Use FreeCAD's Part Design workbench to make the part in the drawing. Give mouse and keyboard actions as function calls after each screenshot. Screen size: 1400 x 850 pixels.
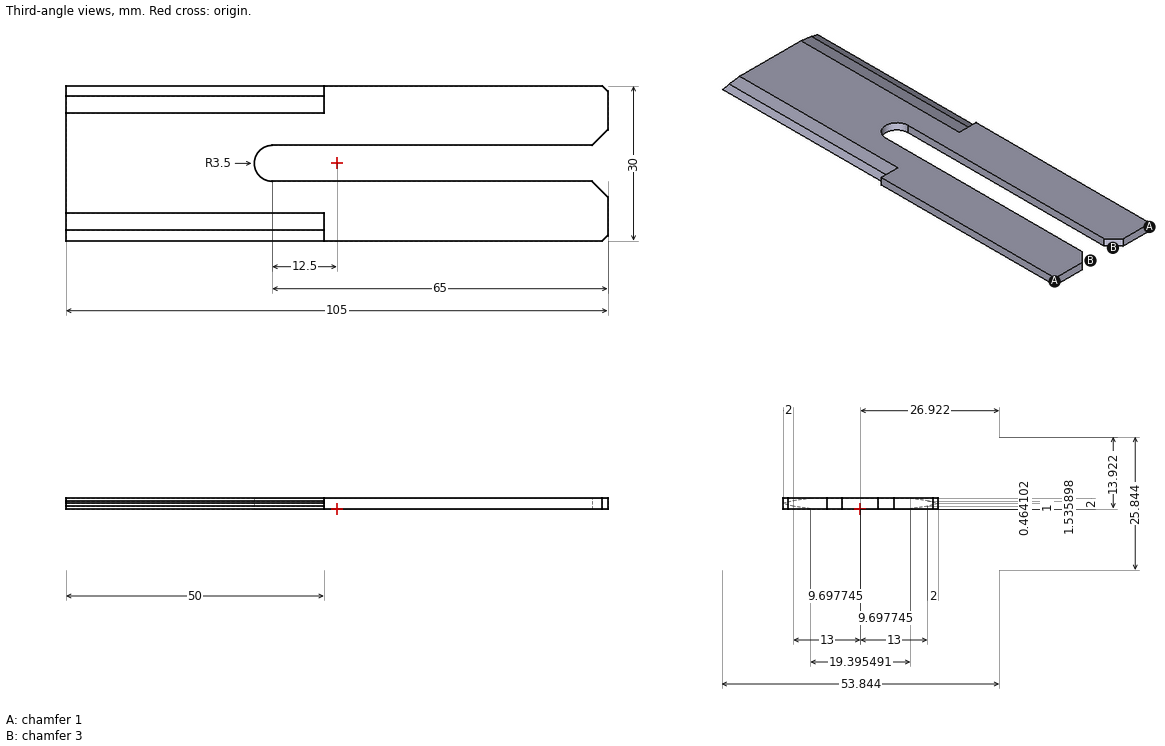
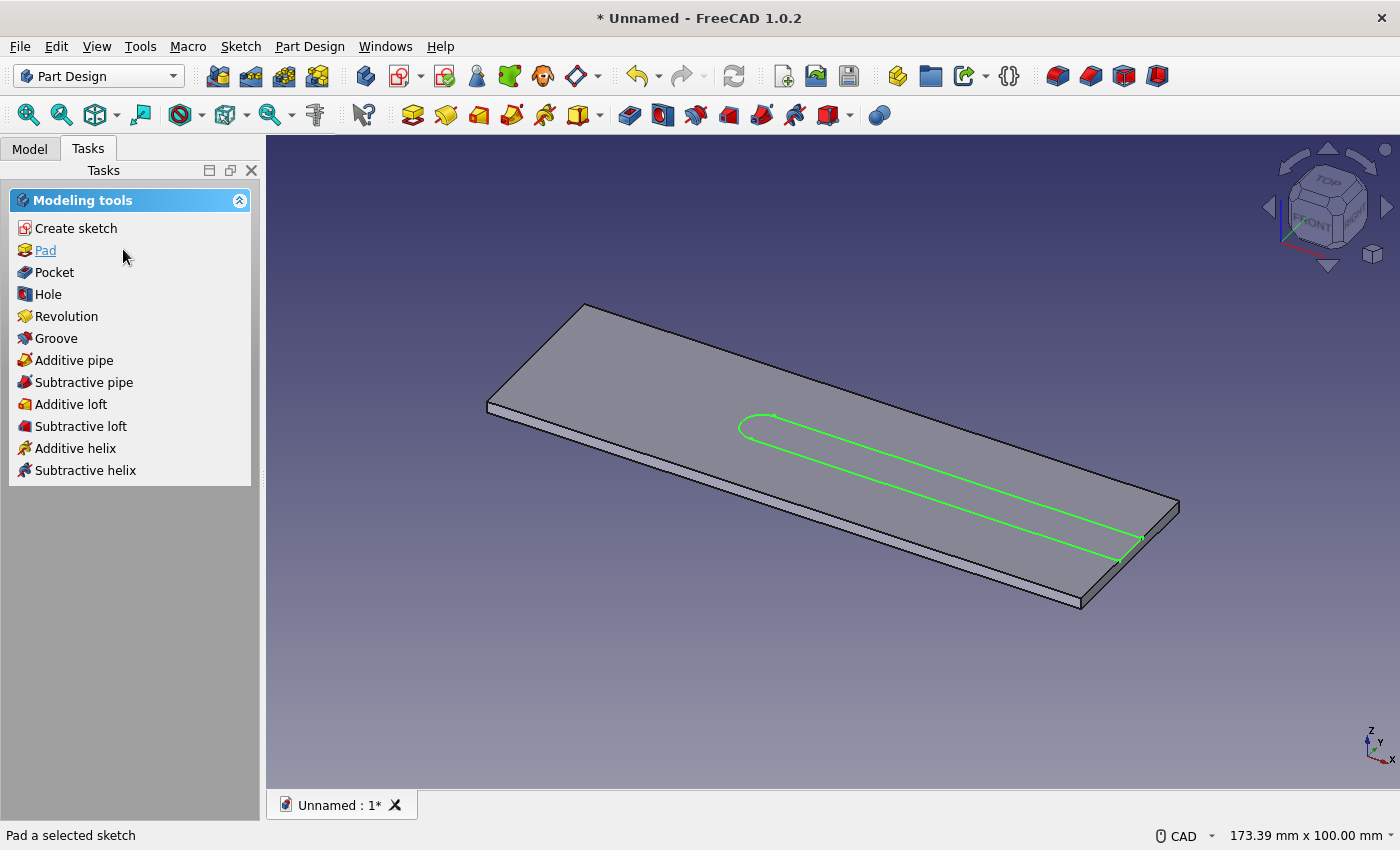
click(630, 116)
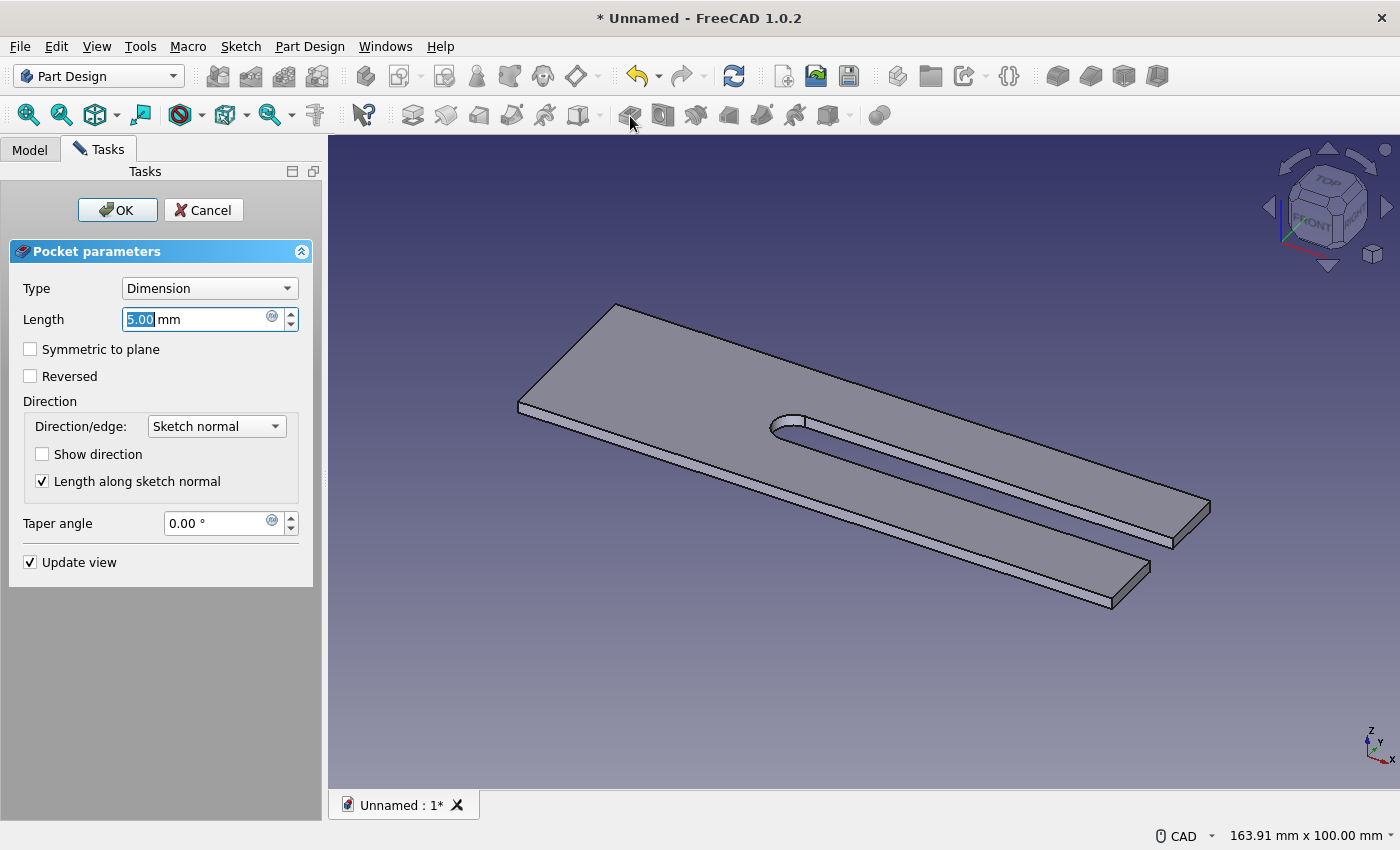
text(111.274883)
key(Tab)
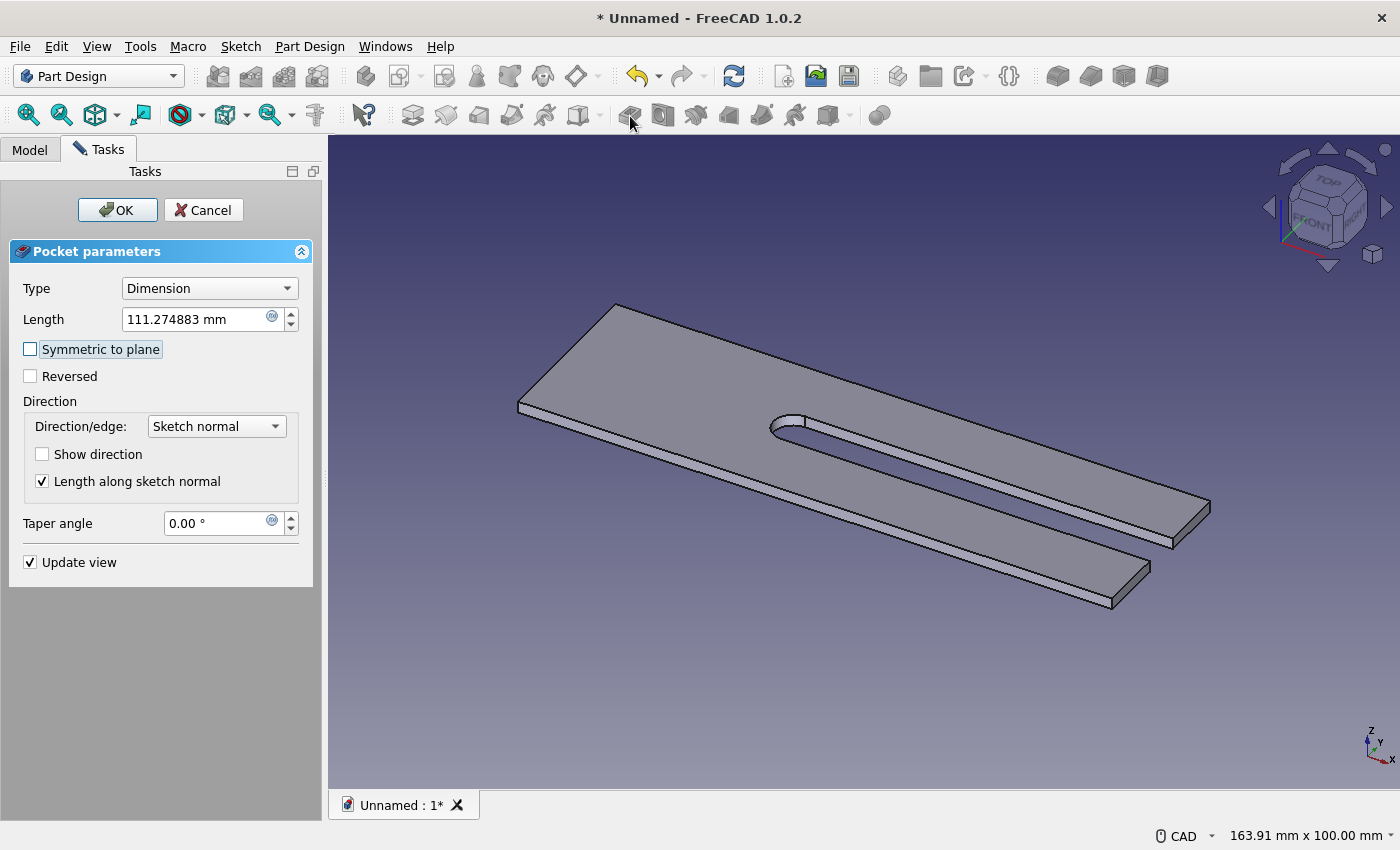
click(31, 349)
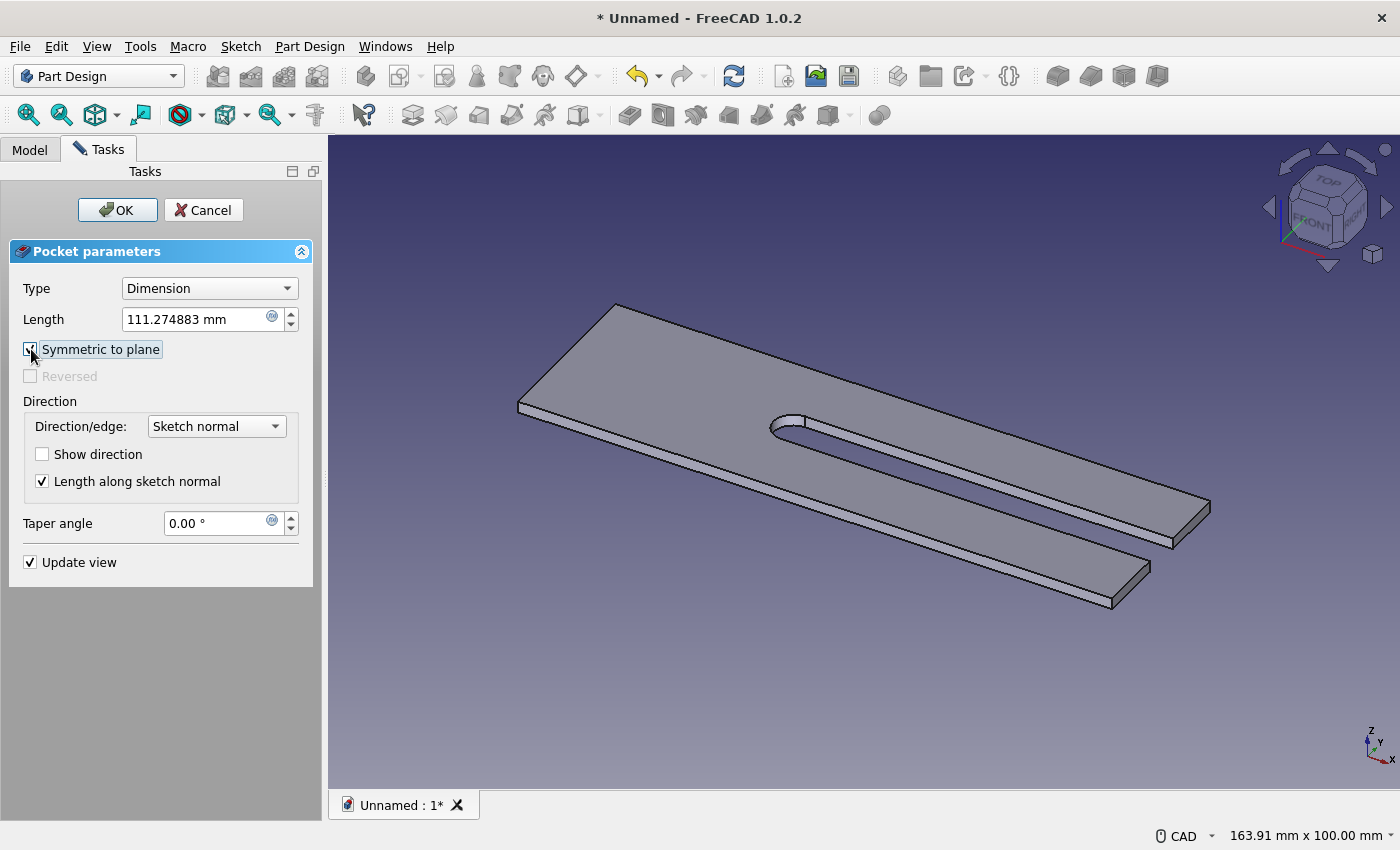
click(118, 210)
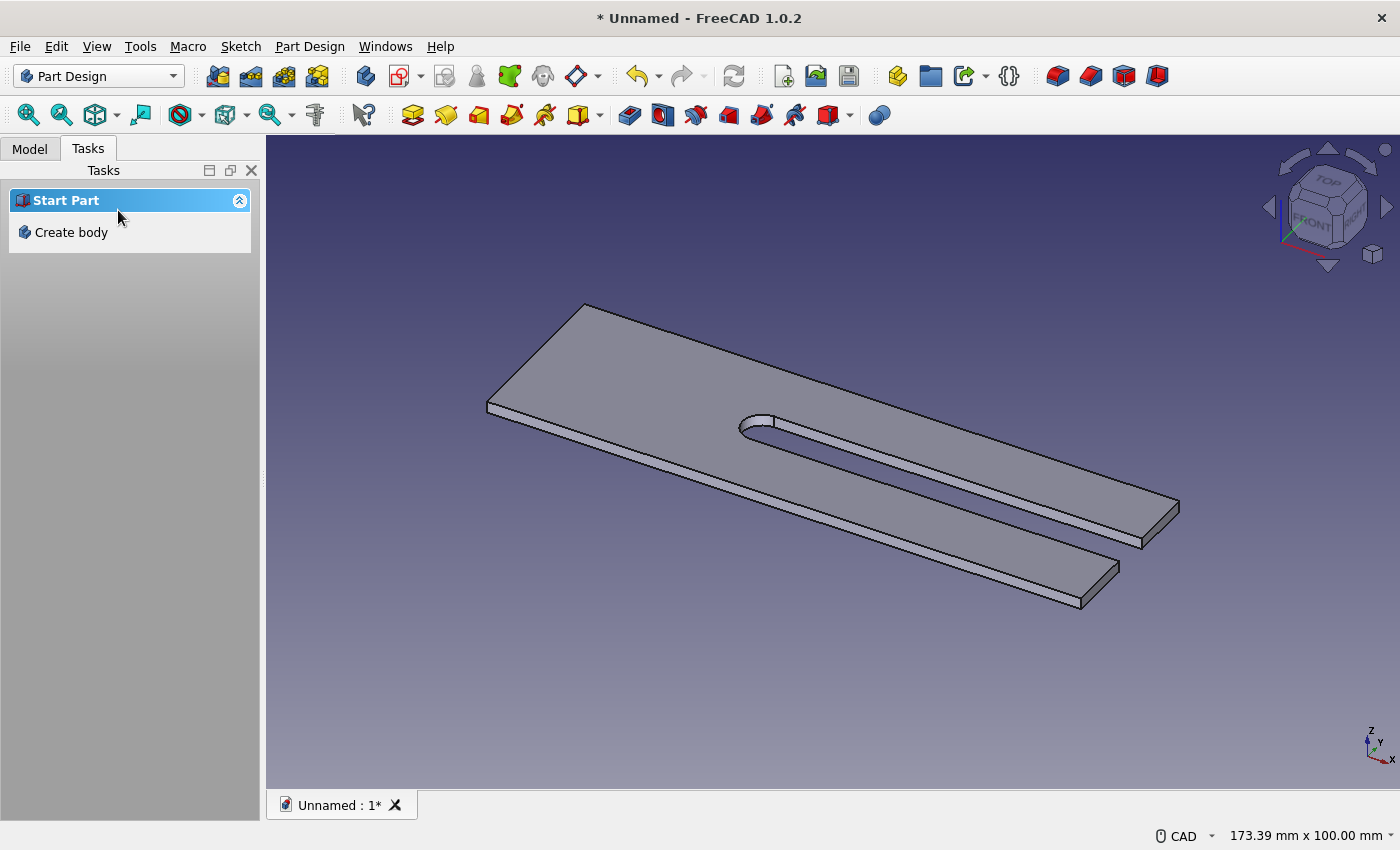
key(6)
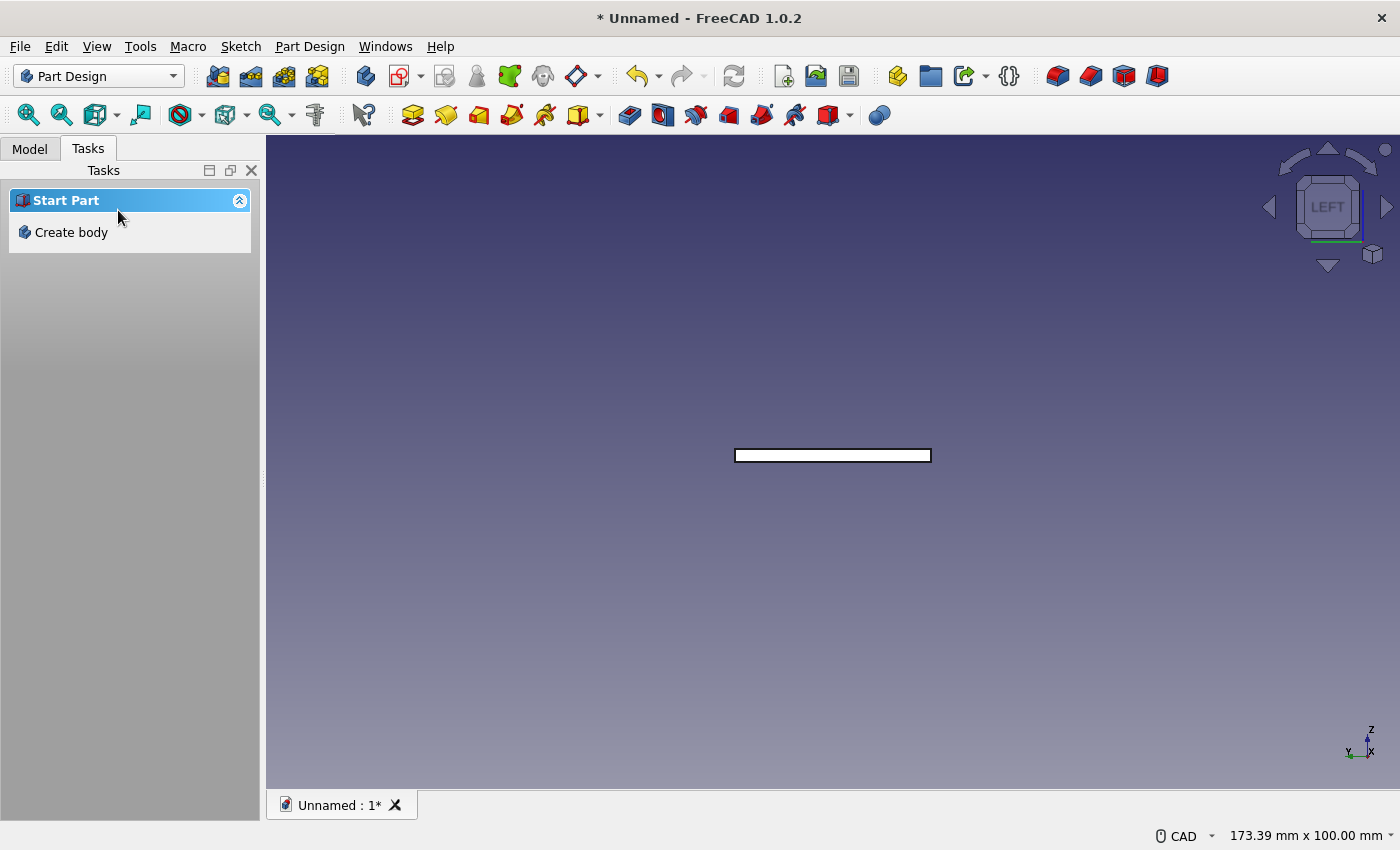
click(29, 116)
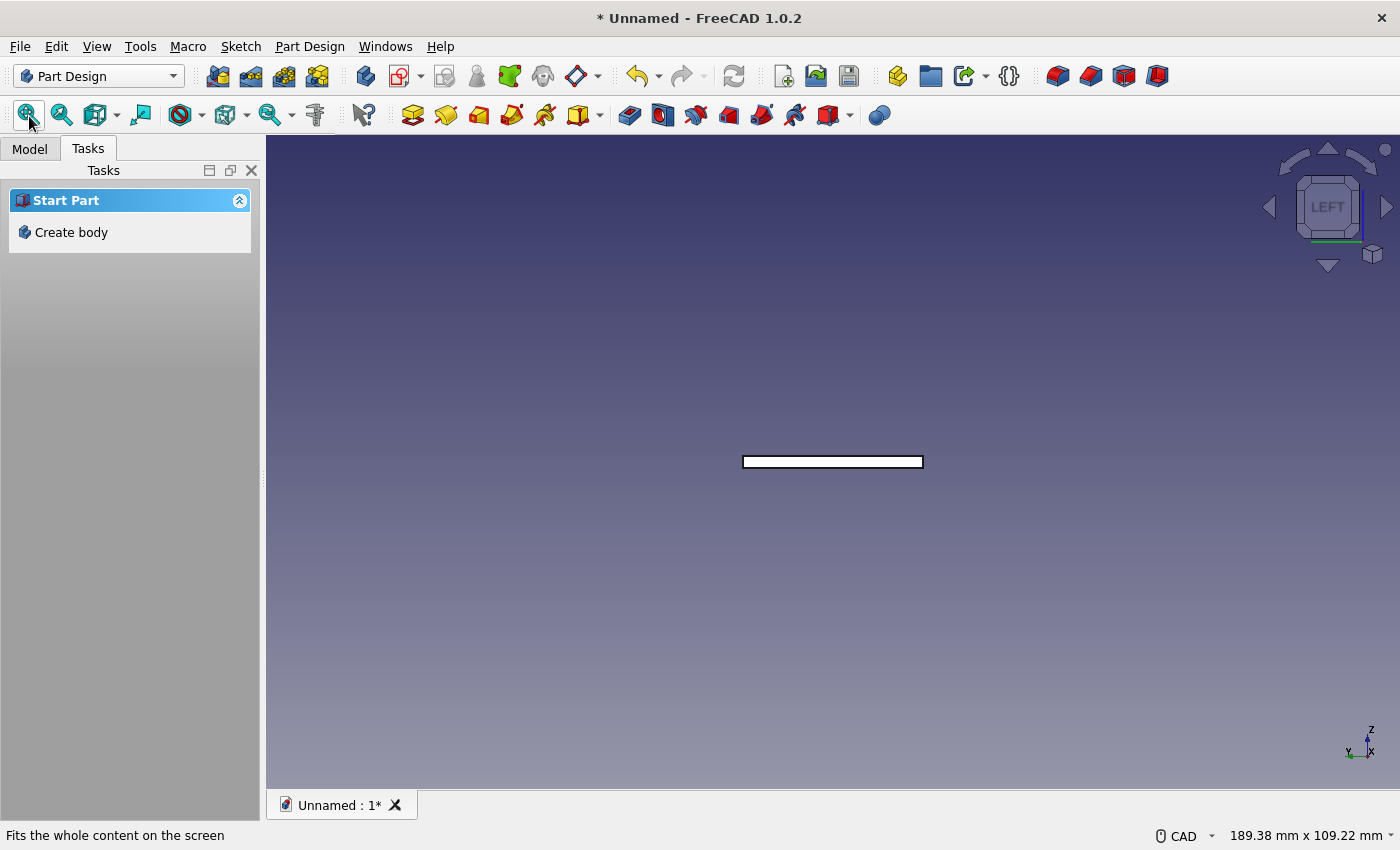
scroll(756, 461, up, 4)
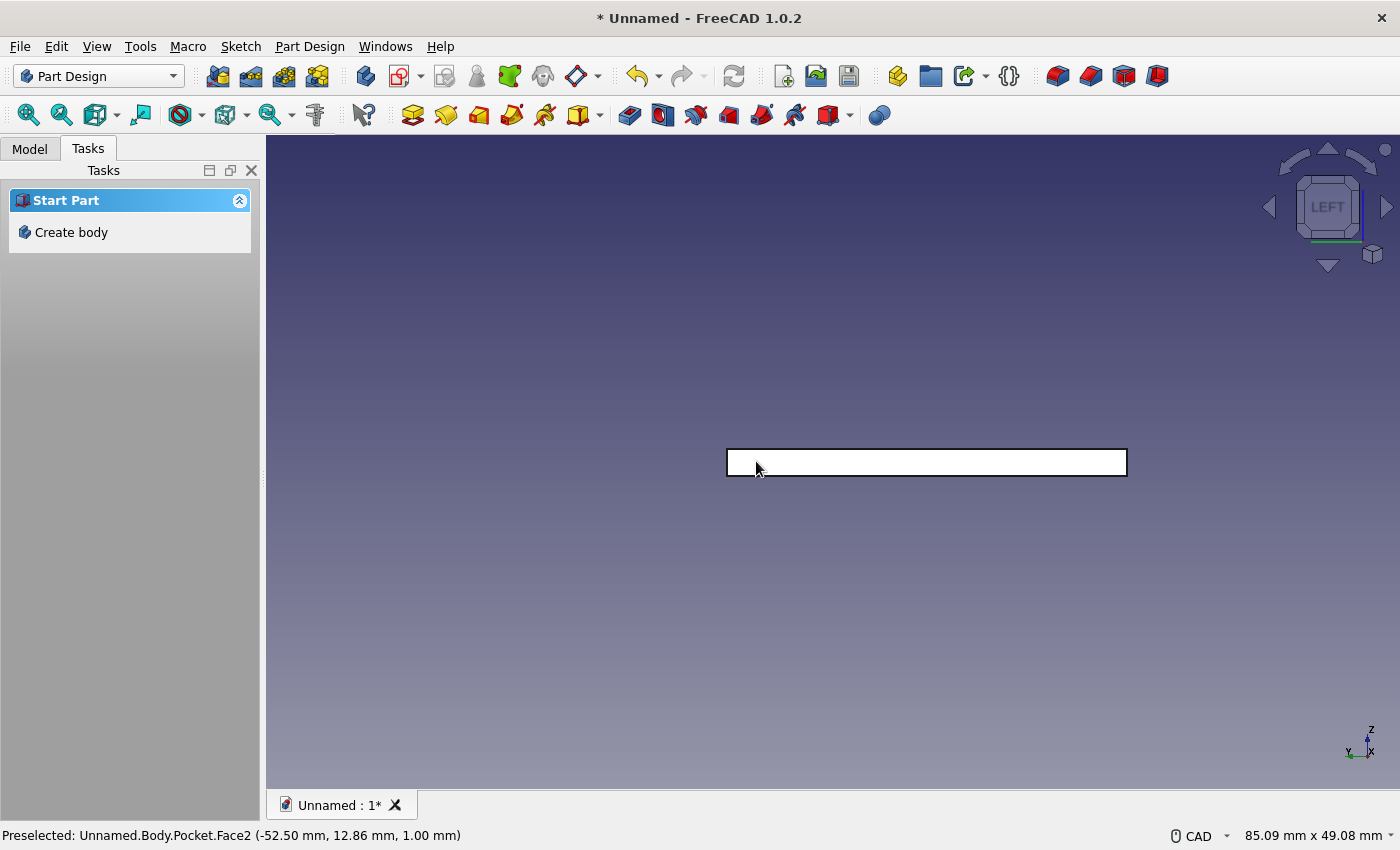
click(755, 462)